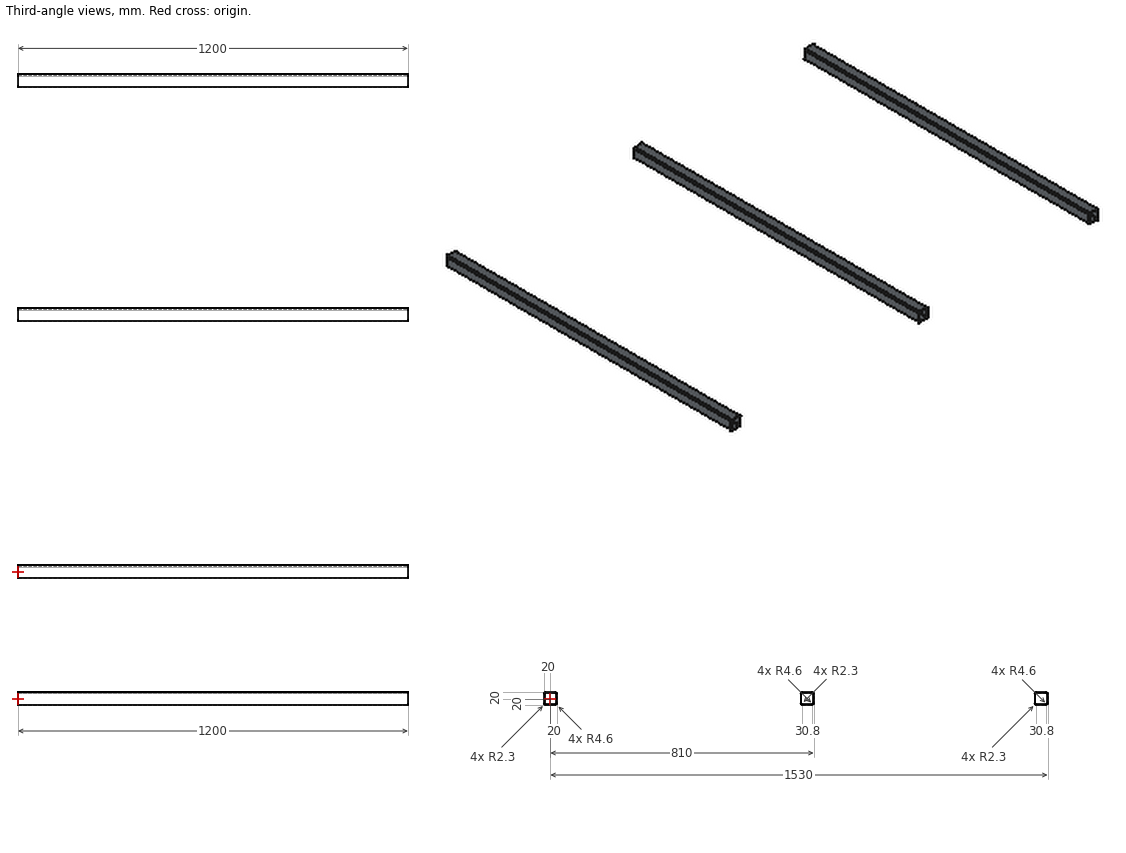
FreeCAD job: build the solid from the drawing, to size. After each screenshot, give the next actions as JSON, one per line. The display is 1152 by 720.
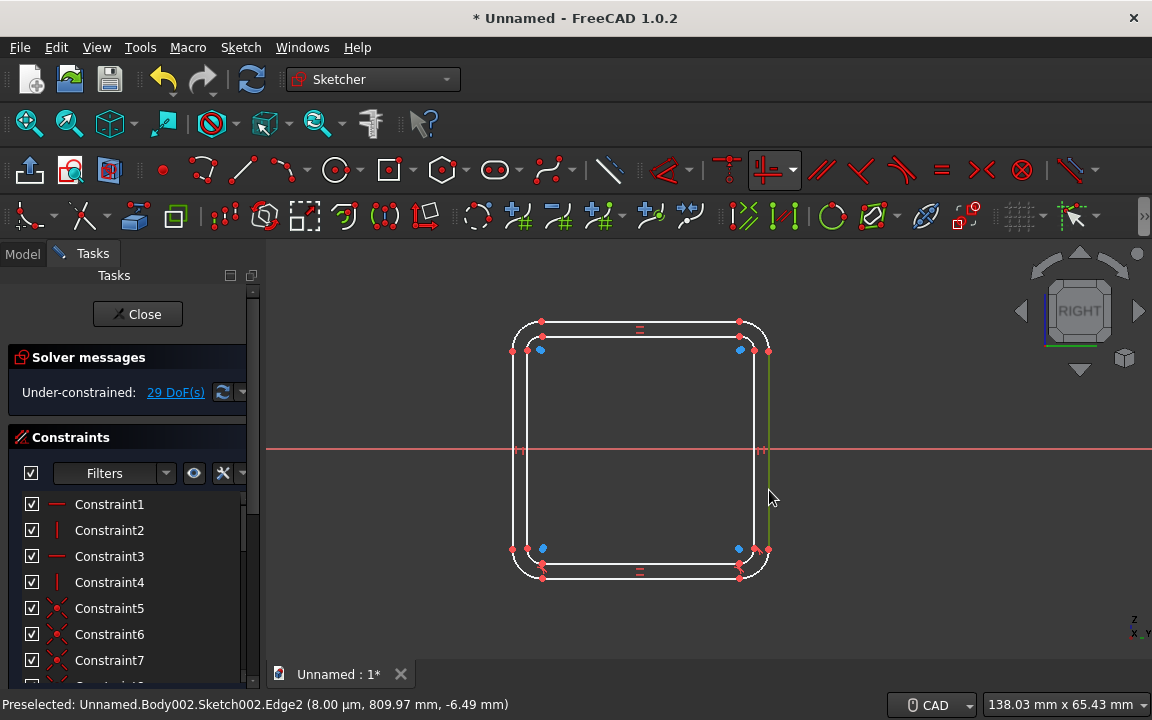
{"action": "left_click", "coordinate": [766, 338]}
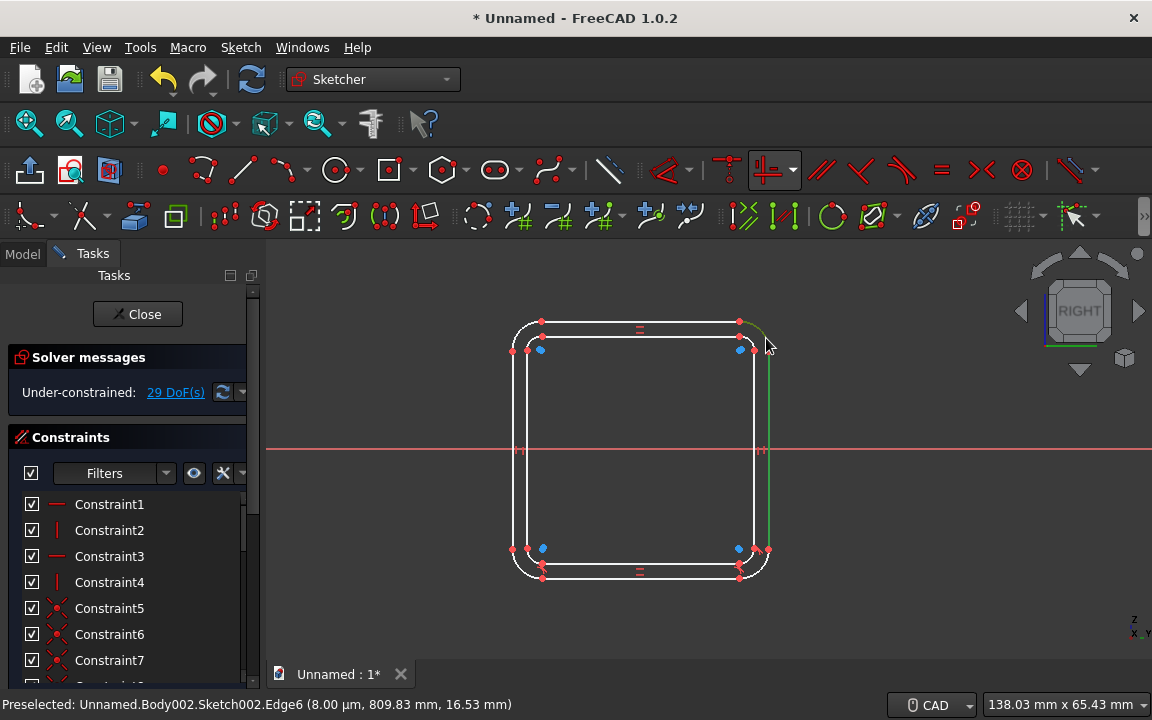
{"action": "key", "text": "t"}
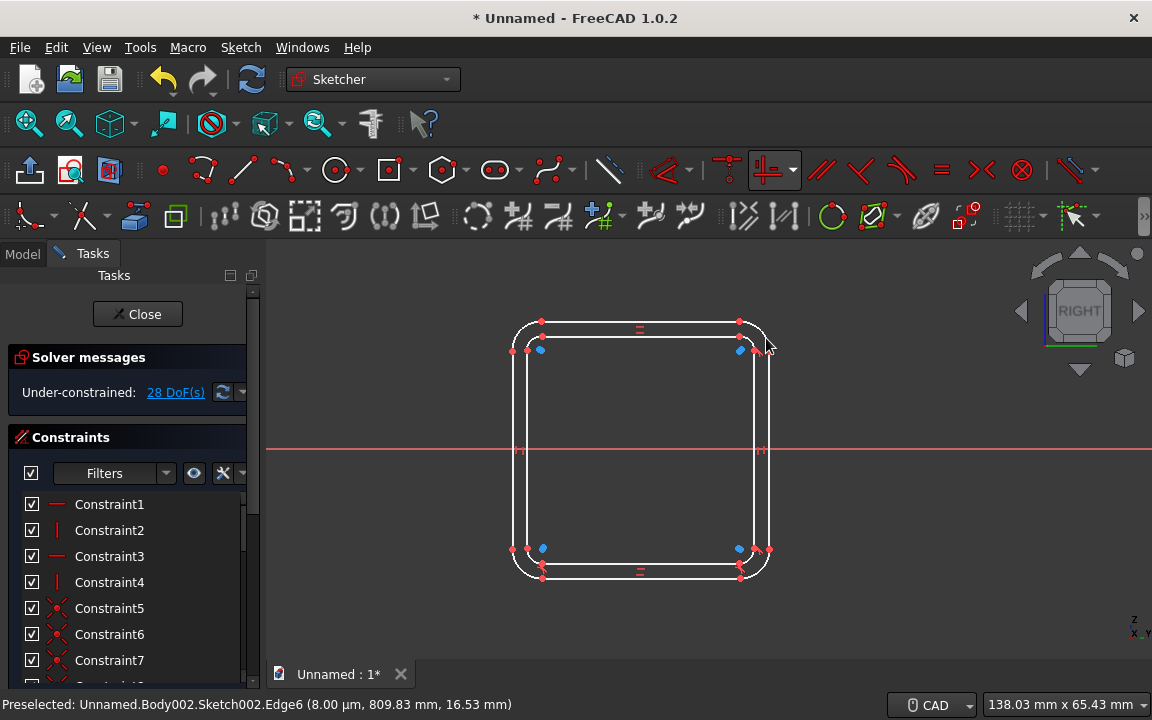
{"action": "left_click", "coordinate": [680, 322]}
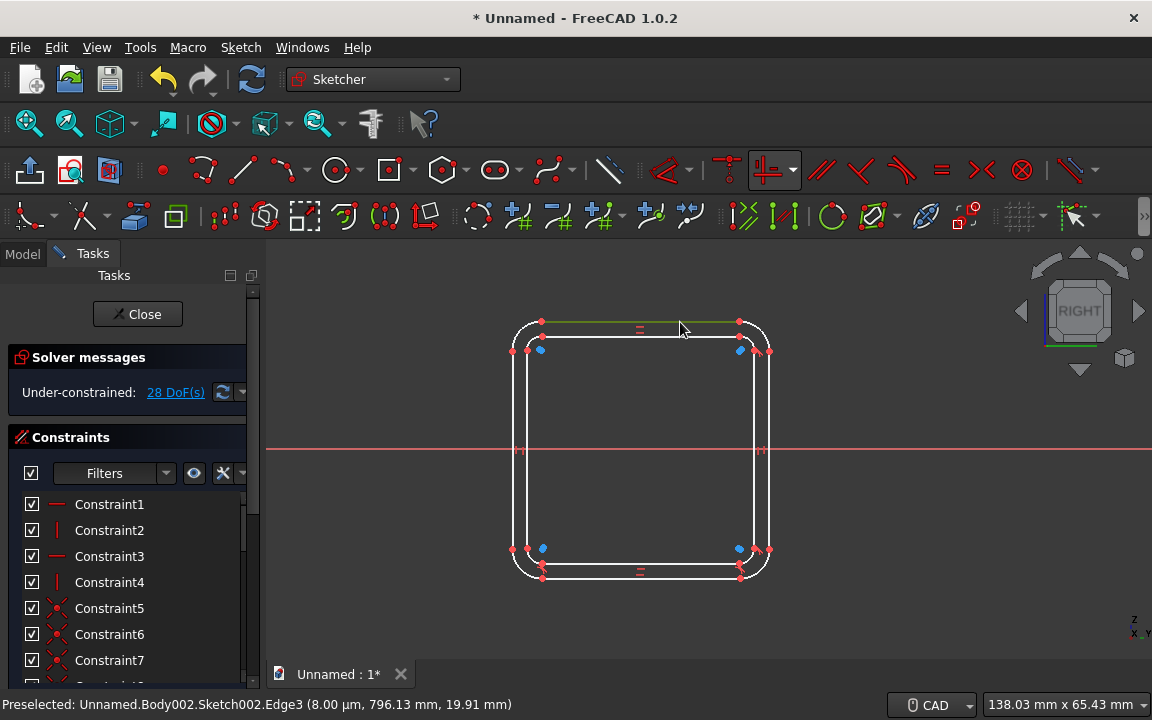
{"action": "left_click", "coordinate": [766, 338]}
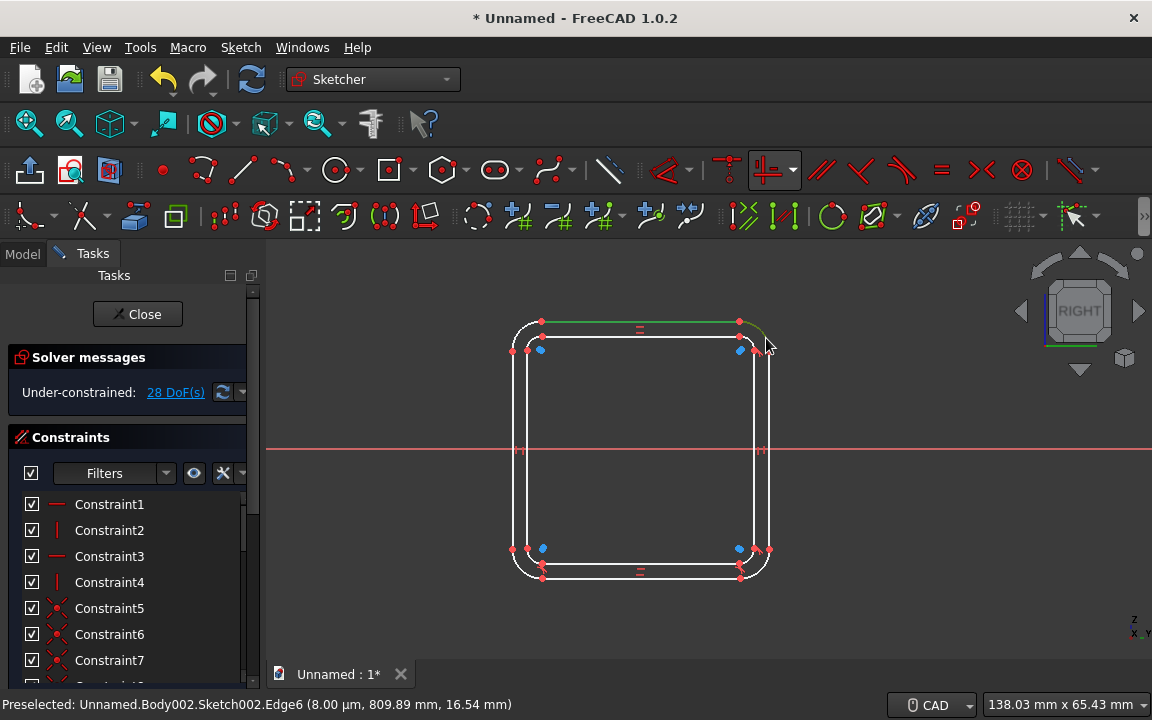
{"action": "key", "text": "t"}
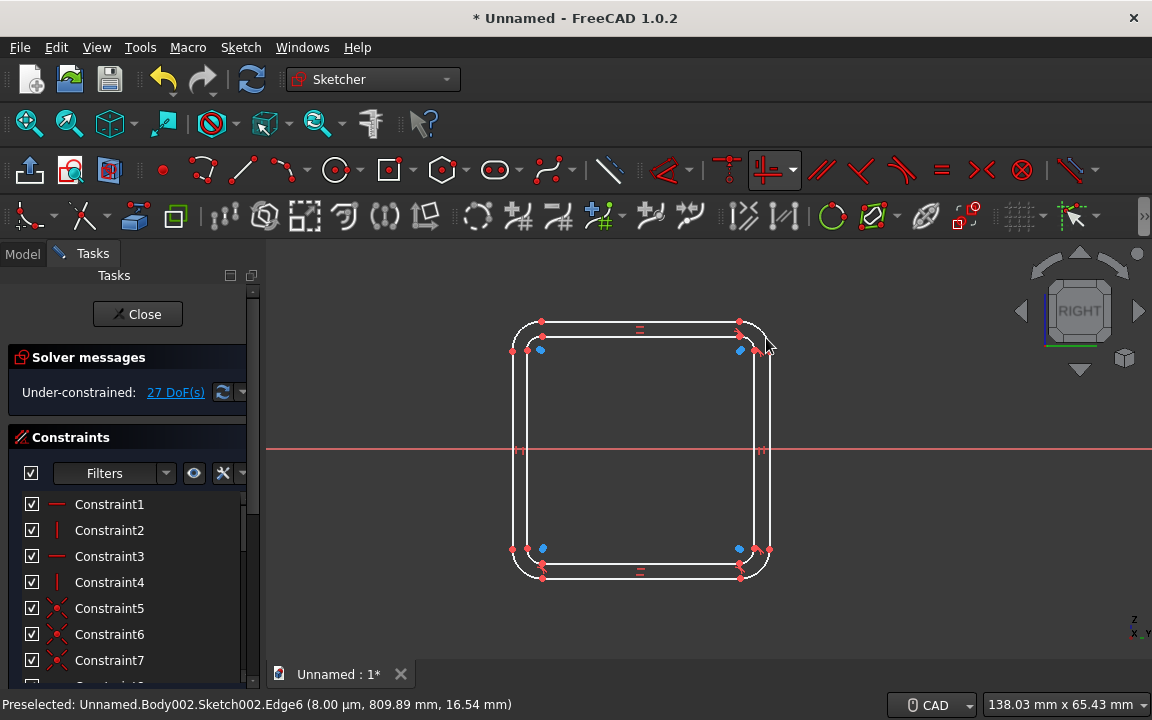
{"action": "left_click", "coordinate": [680, 322]}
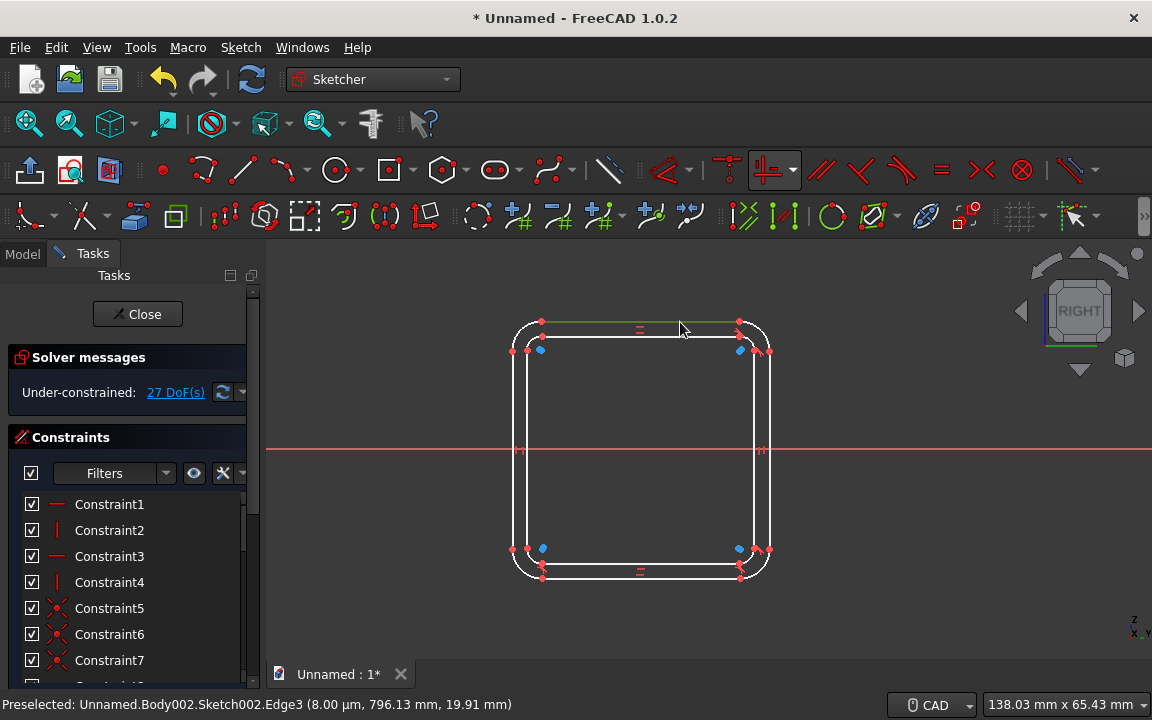
{"action": "left_click", "coordinate": [528, 325]}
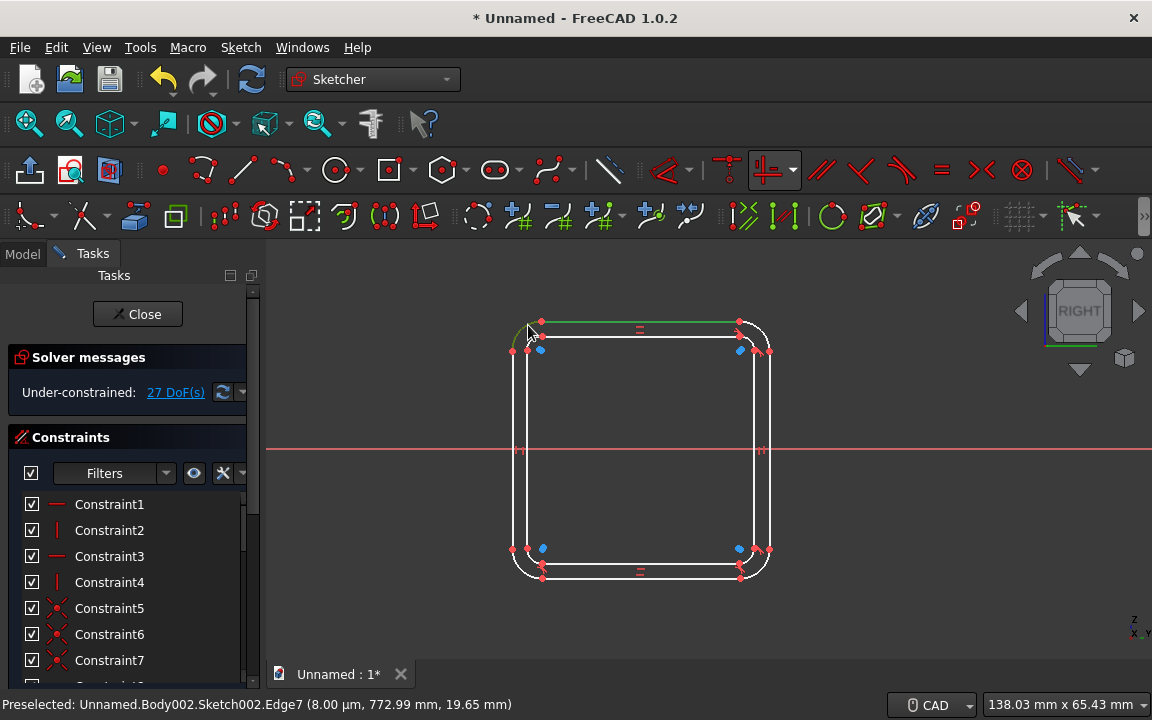
{"action": "key", "text": "t"}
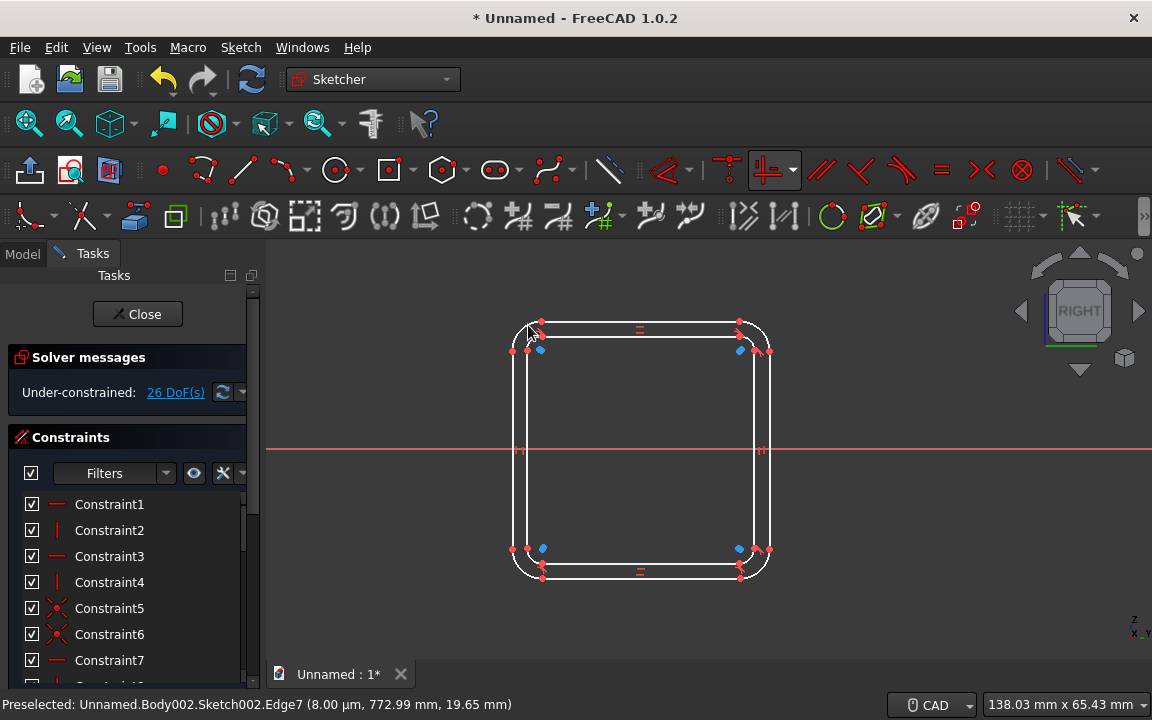
{"action": "left_click", "coordinate": [513, 411]}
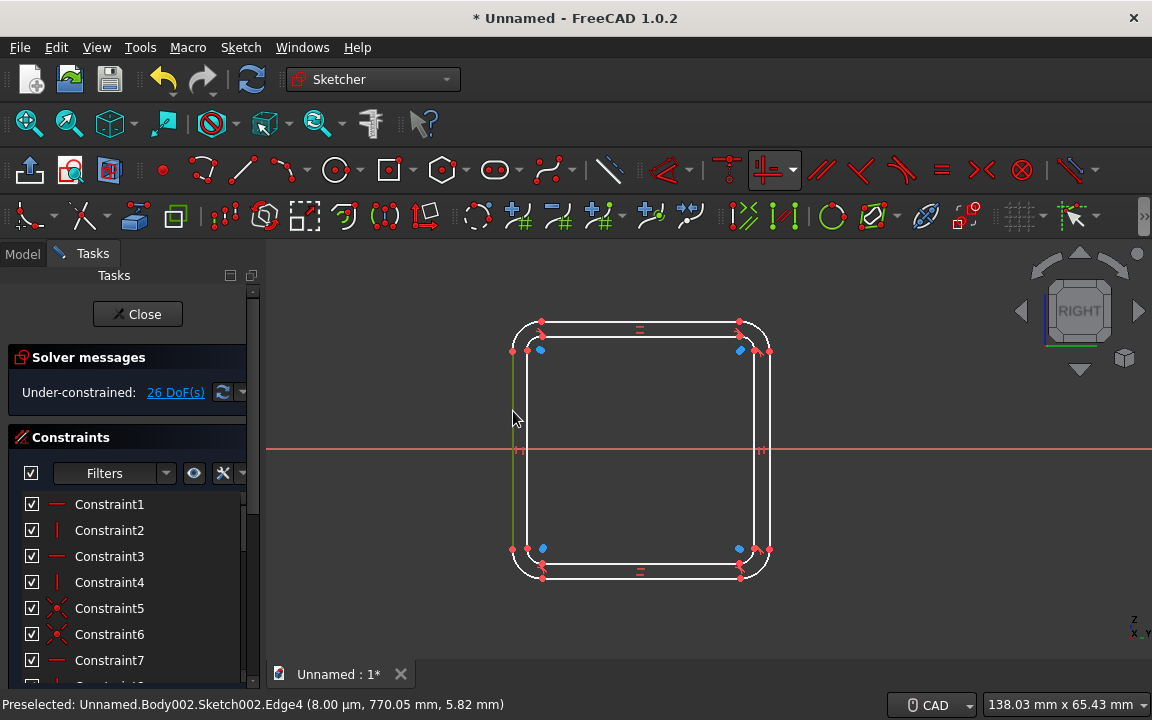
{"action": "left_click", "coordinate": [528, 325]}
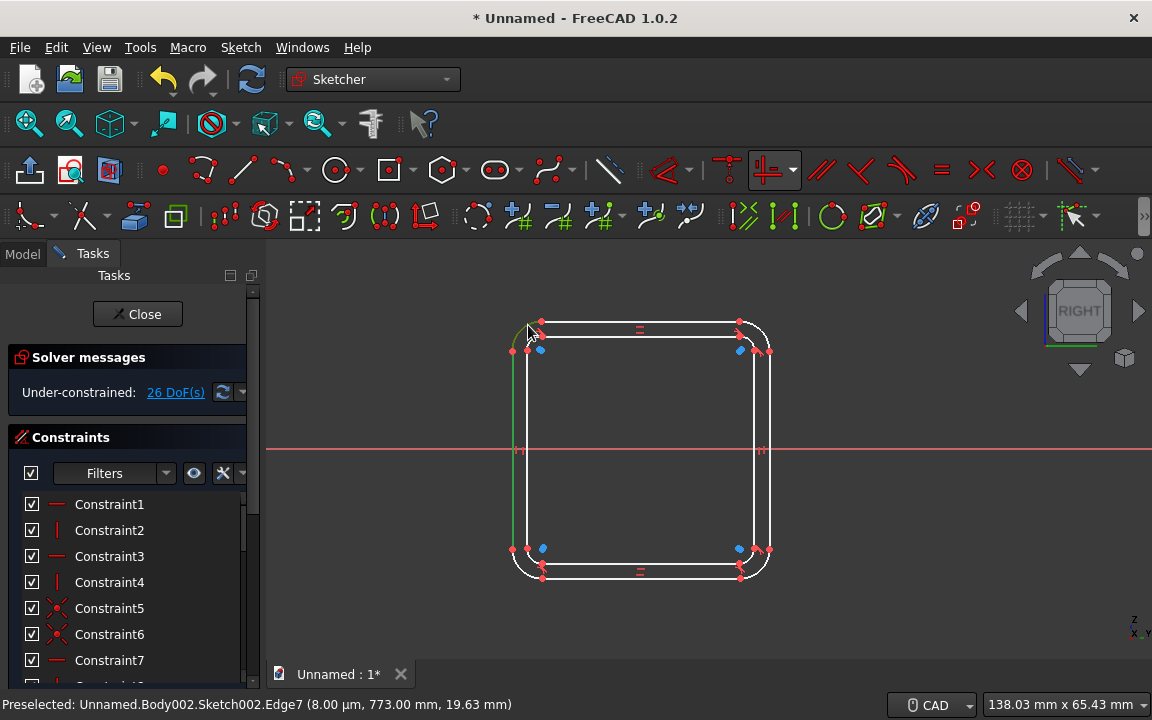
{"action": "key", "text": "t"}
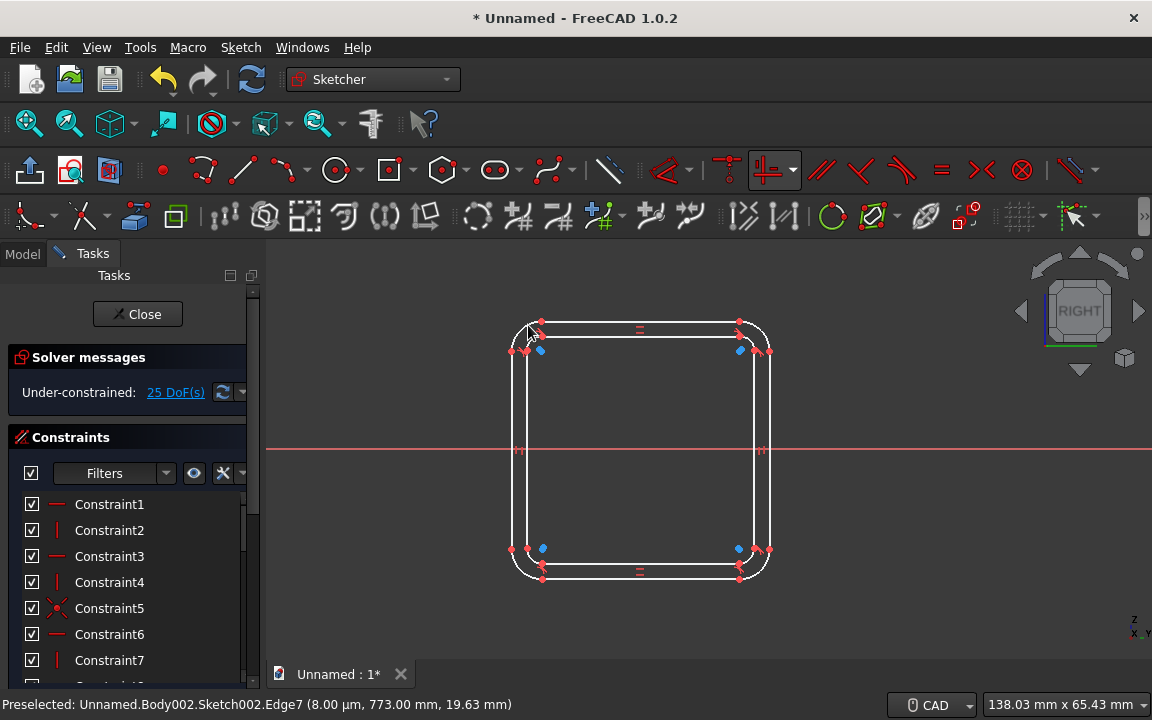
{"action": "left_click", "coordinate": [512, 411]}